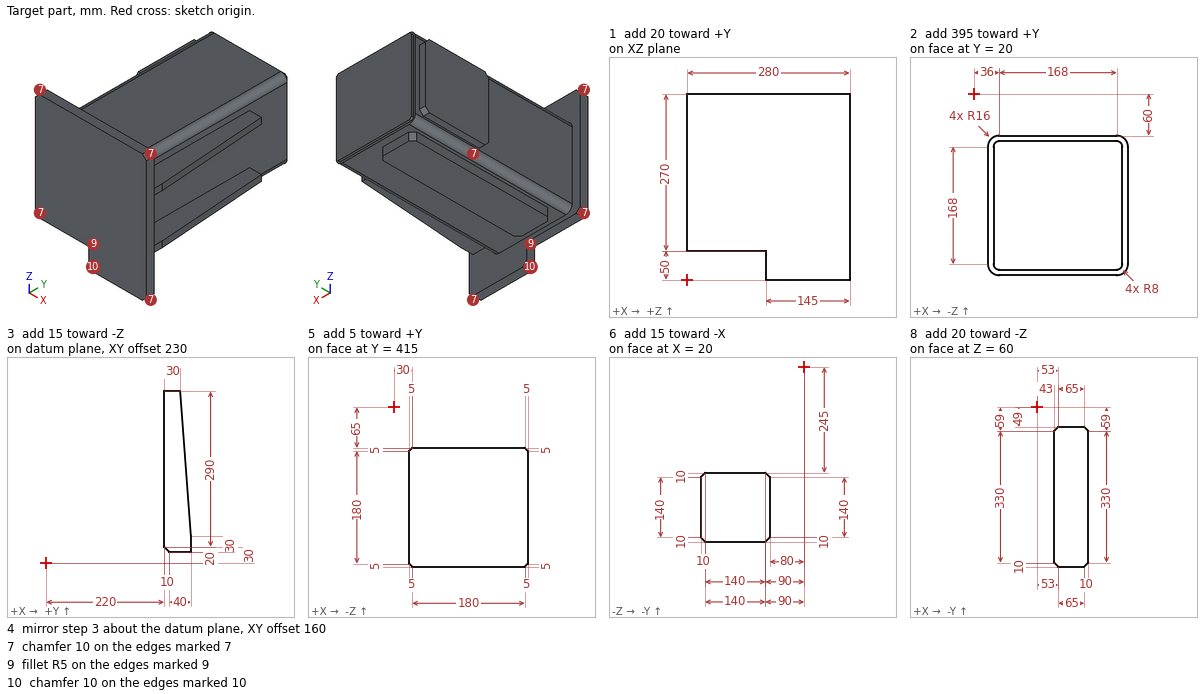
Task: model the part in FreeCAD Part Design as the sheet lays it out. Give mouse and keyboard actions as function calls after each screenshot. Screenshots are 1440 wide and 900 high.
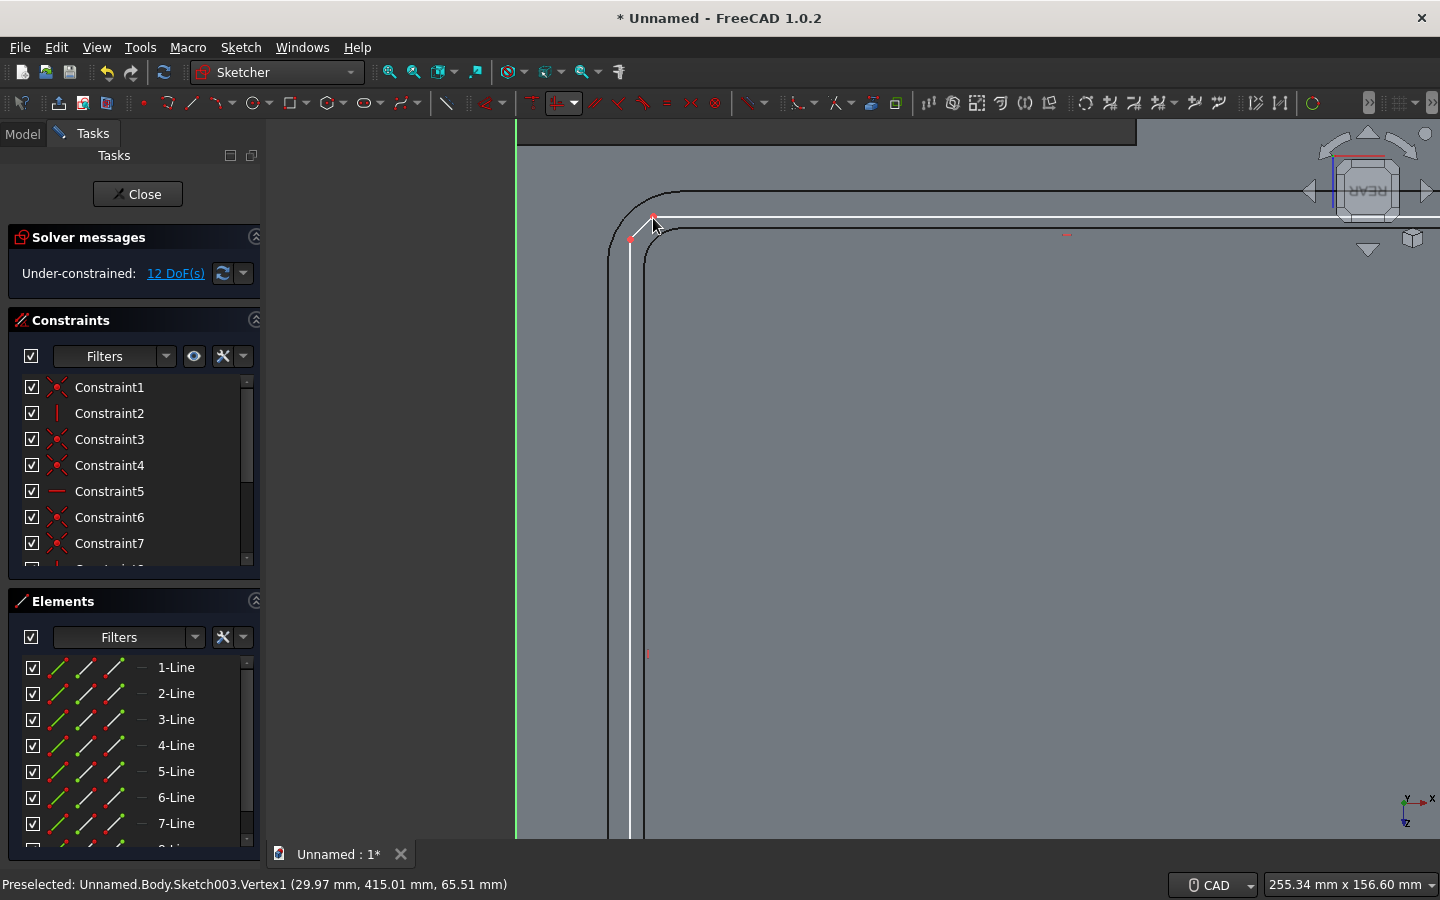
key(d)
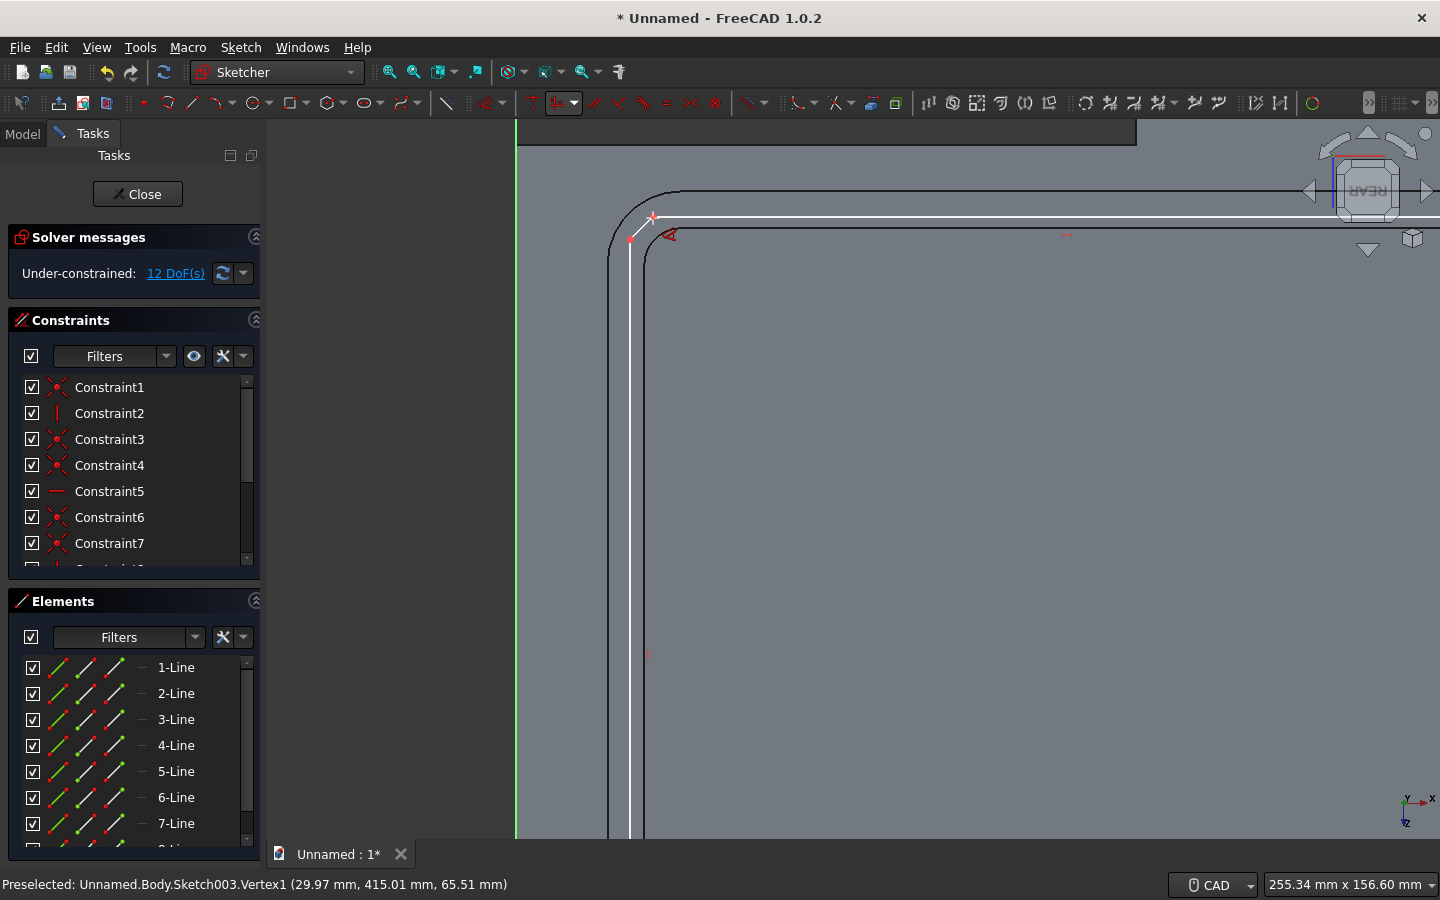
scroll(646, 223, up, 3)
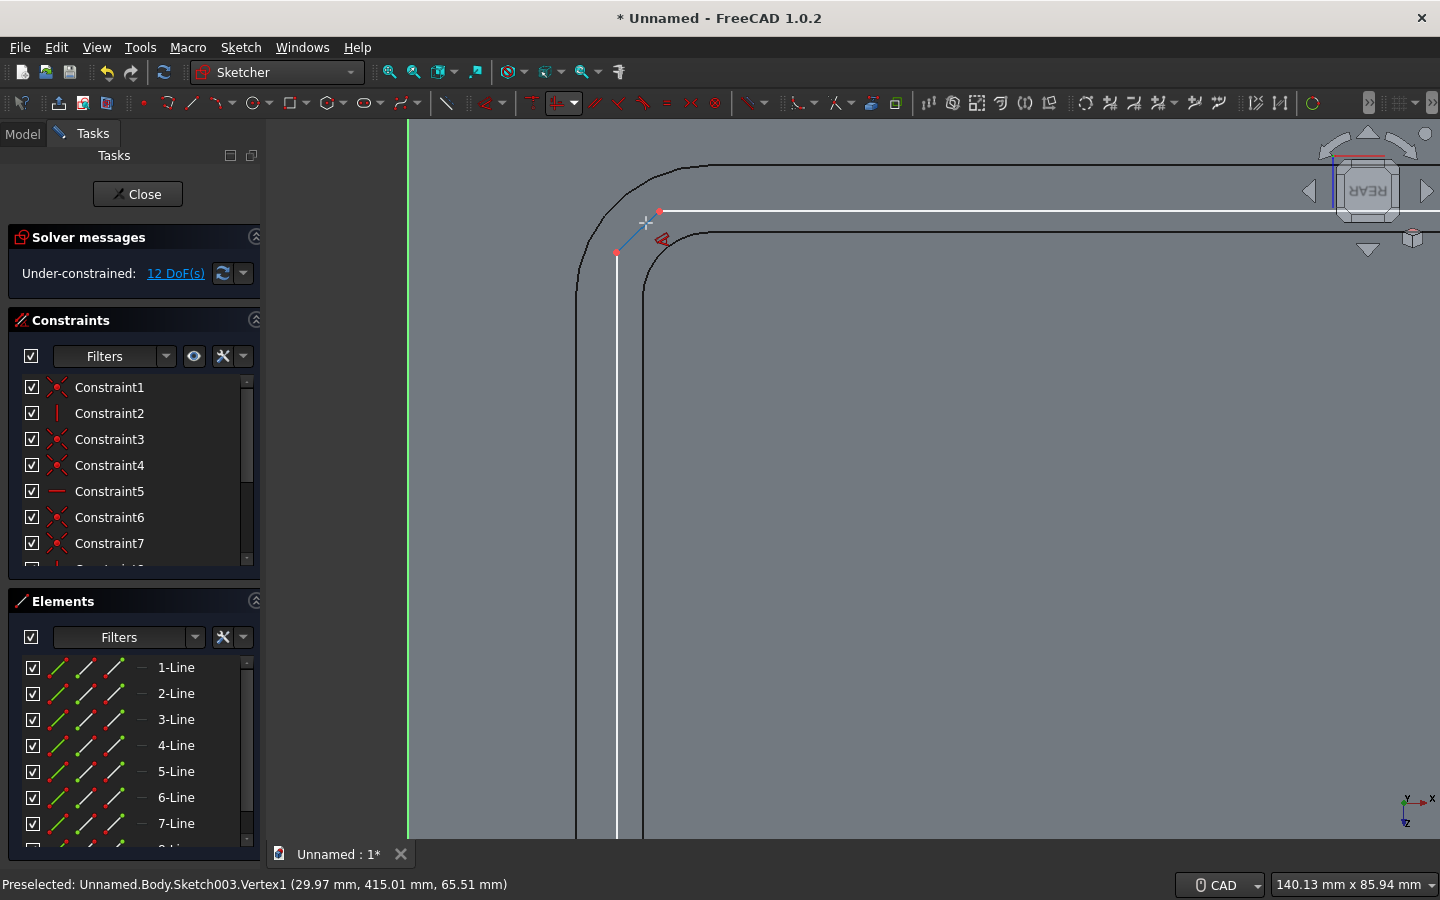
click(646, 224)
click(638, 177)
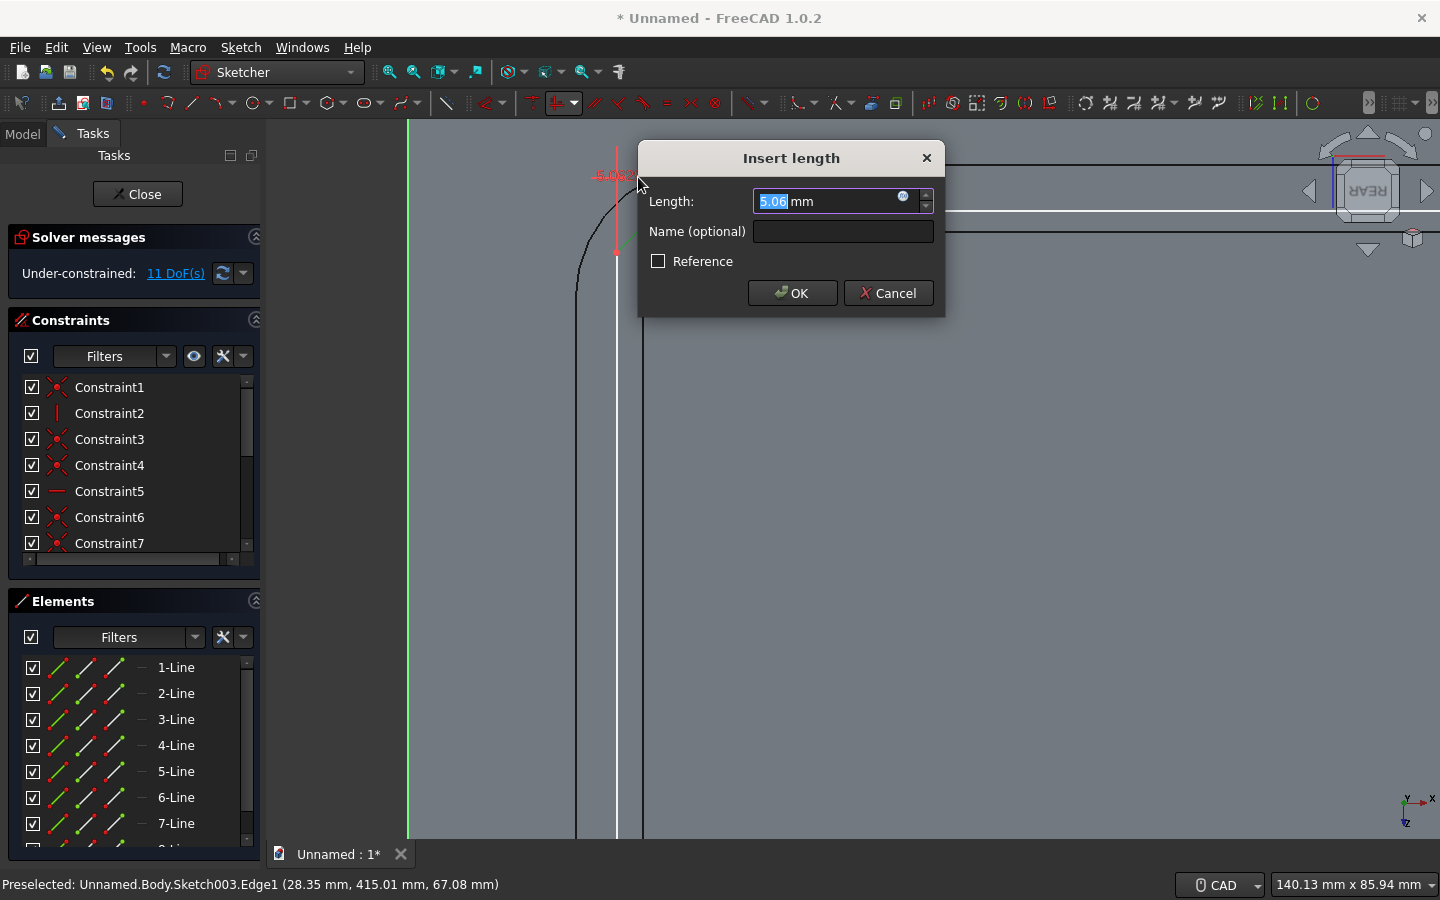
text(5)
key(Return)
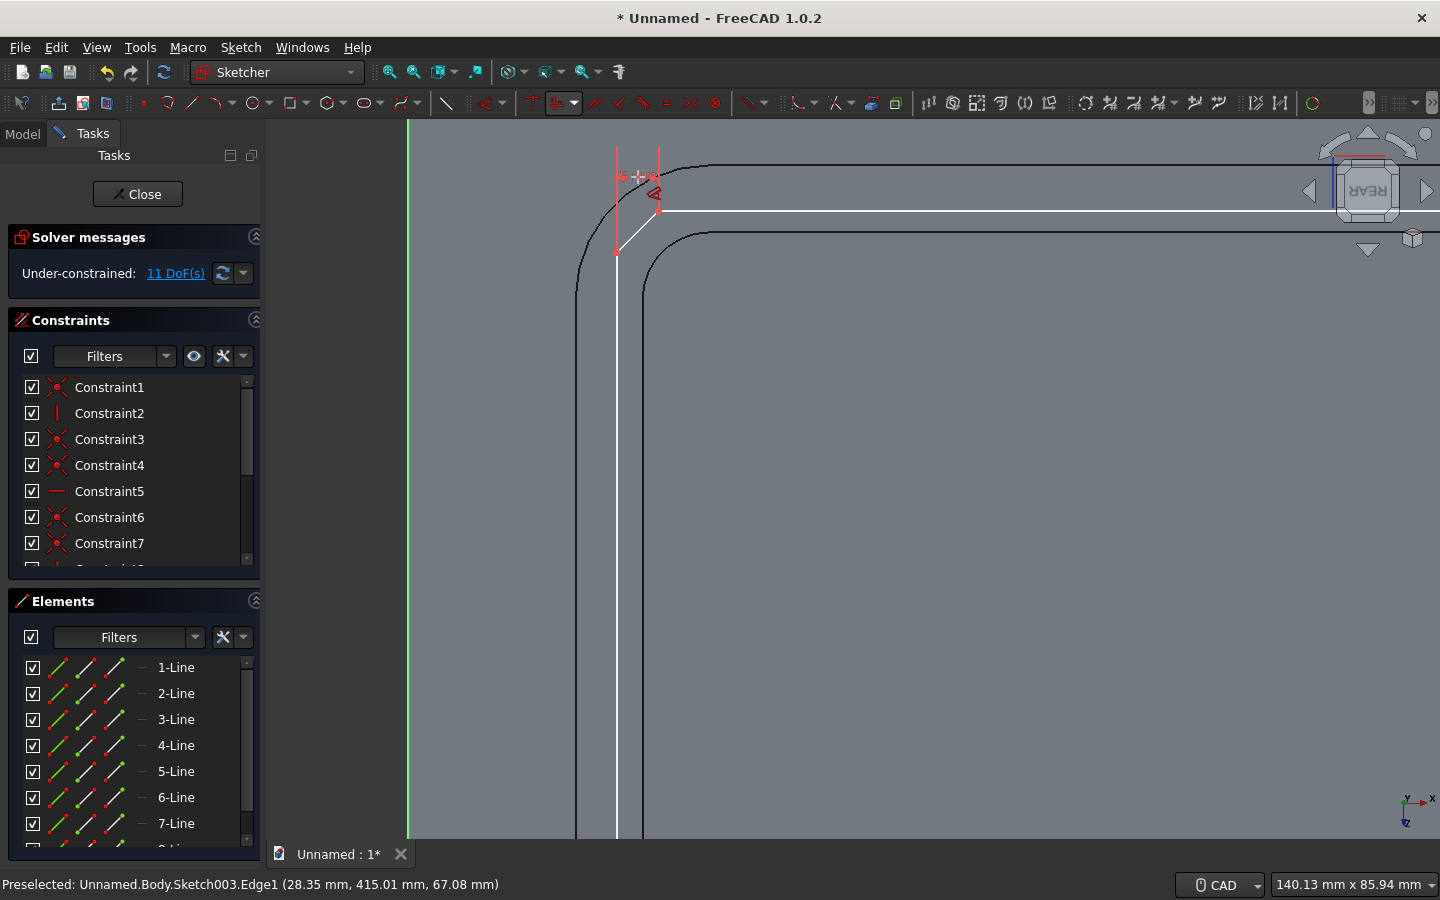
click(646, 224)
click(583, 232)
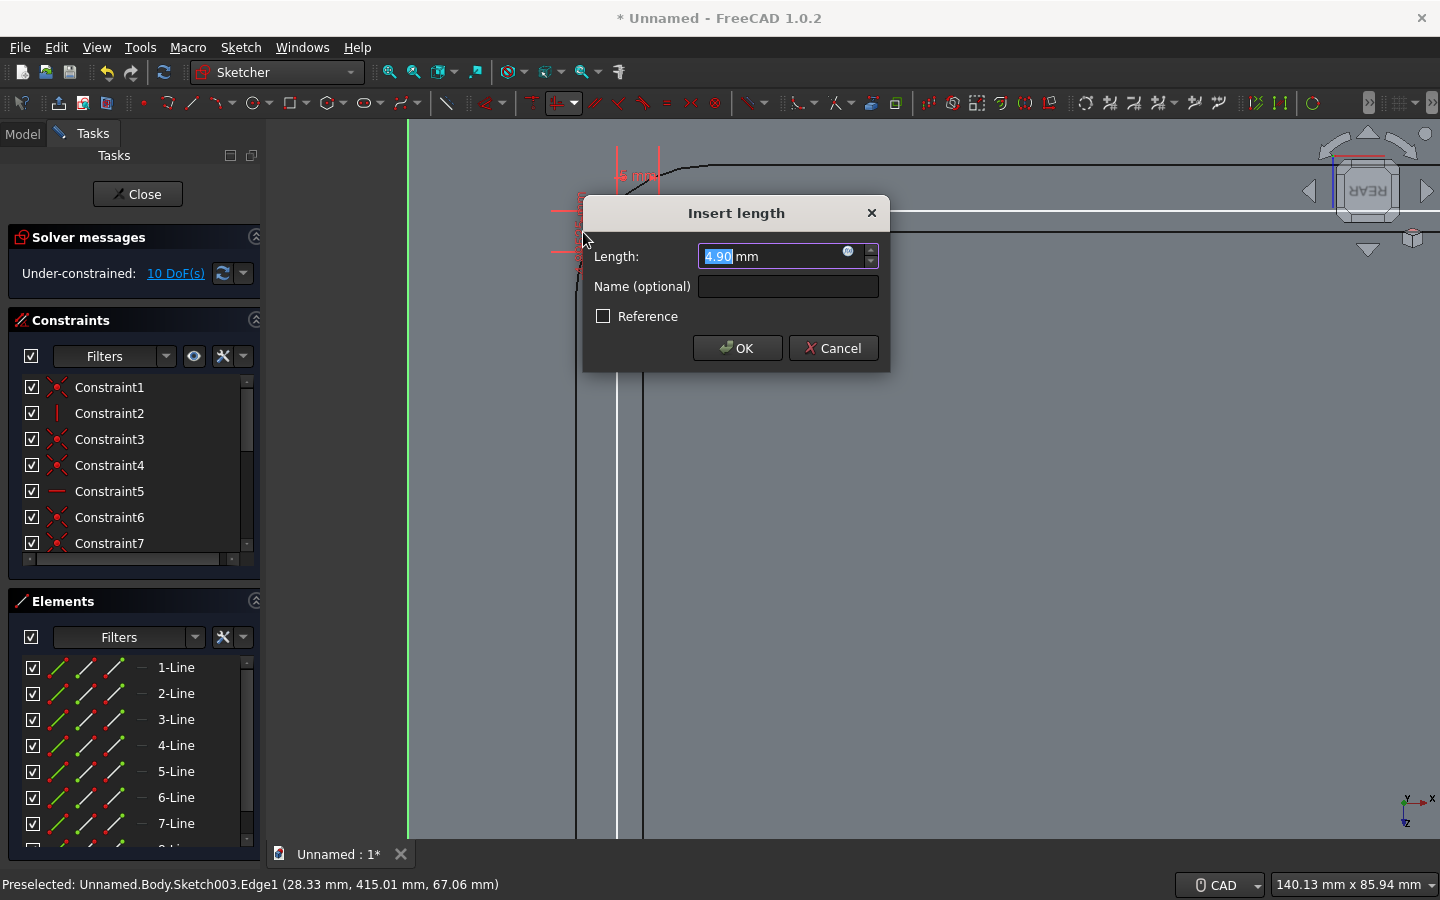
text(5)
key(Return)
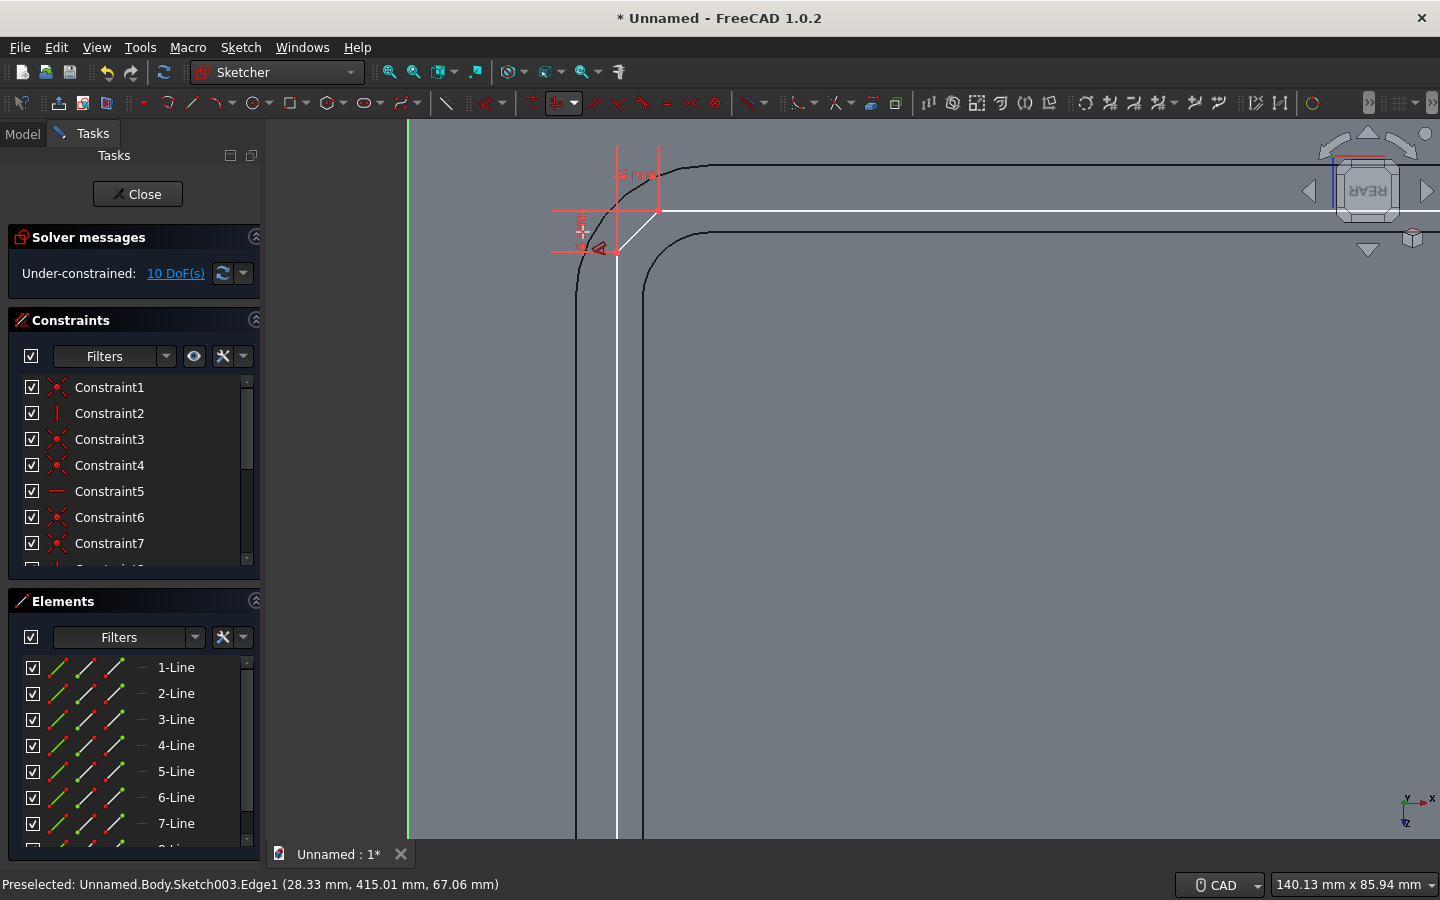
scroll(652, 415, down, 8)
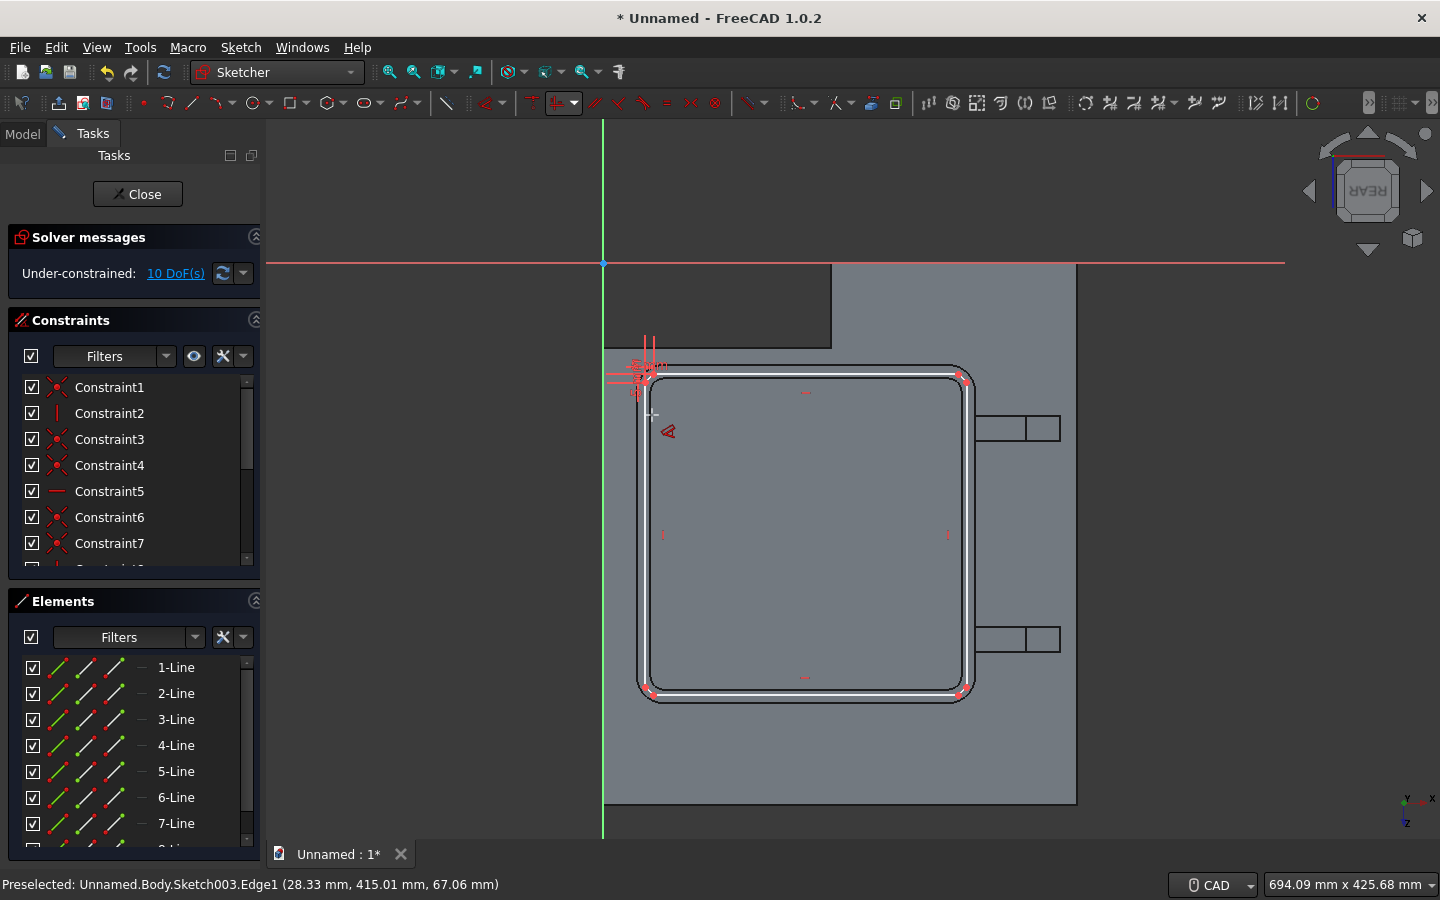
scroll(648, 690, up, 8)